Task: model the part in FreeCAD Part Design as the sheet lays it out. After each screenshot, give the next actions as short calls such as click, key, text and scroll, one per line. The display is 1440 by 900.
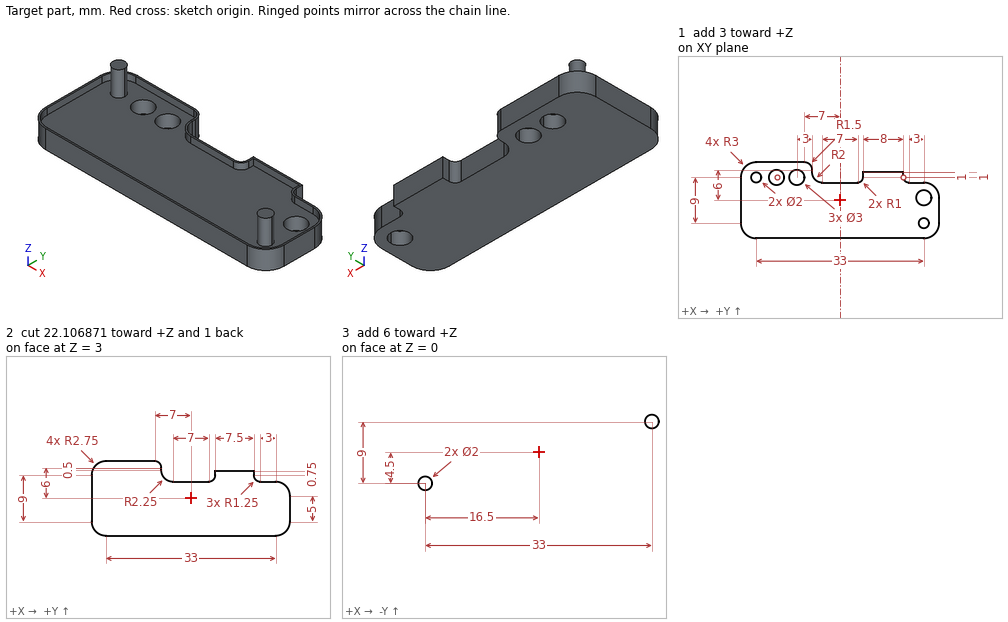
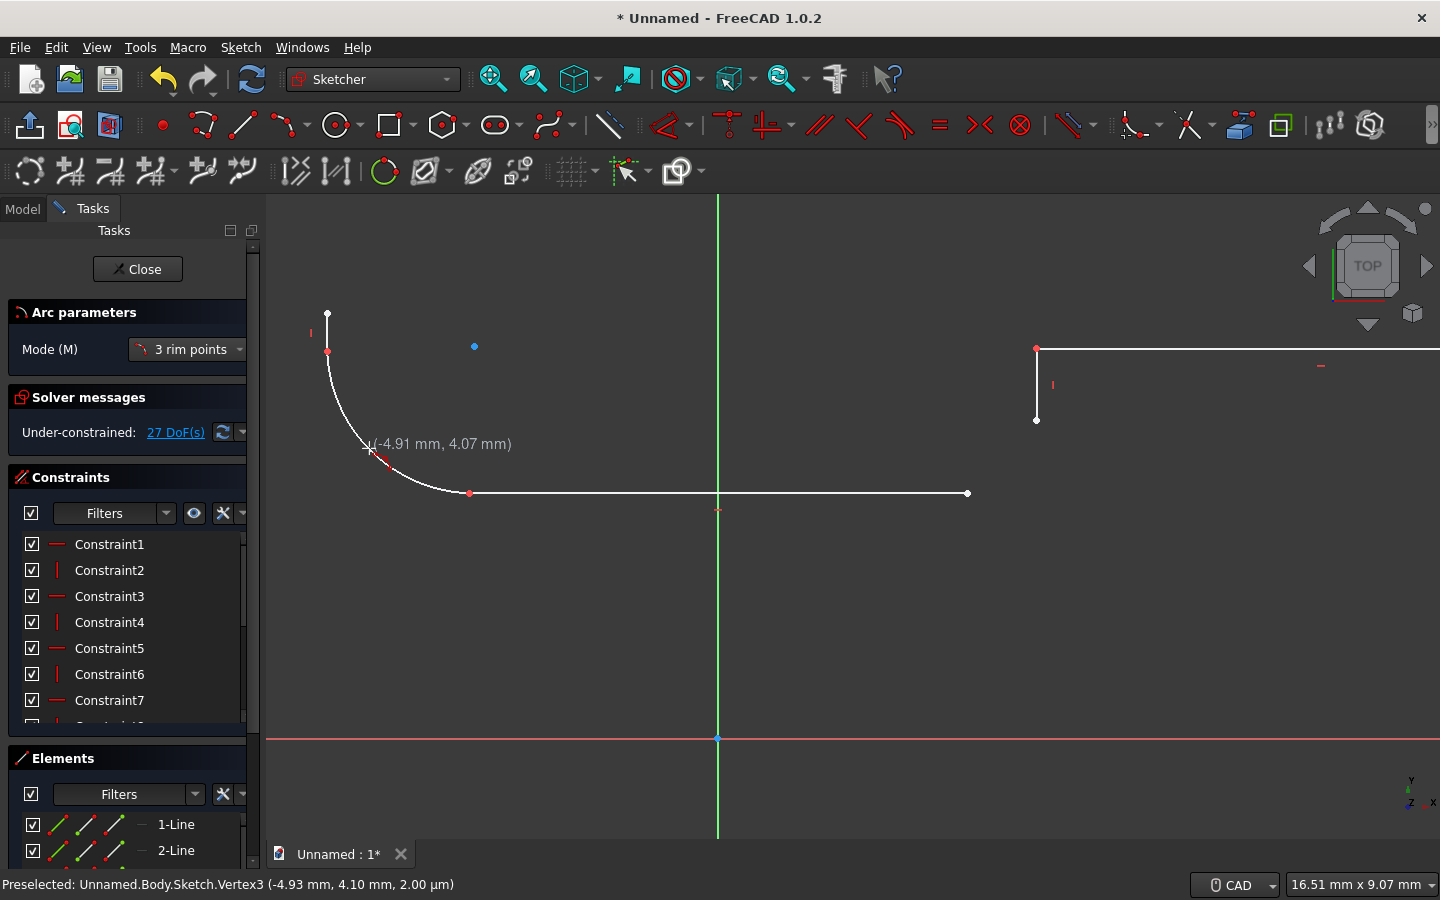
click(327, 314)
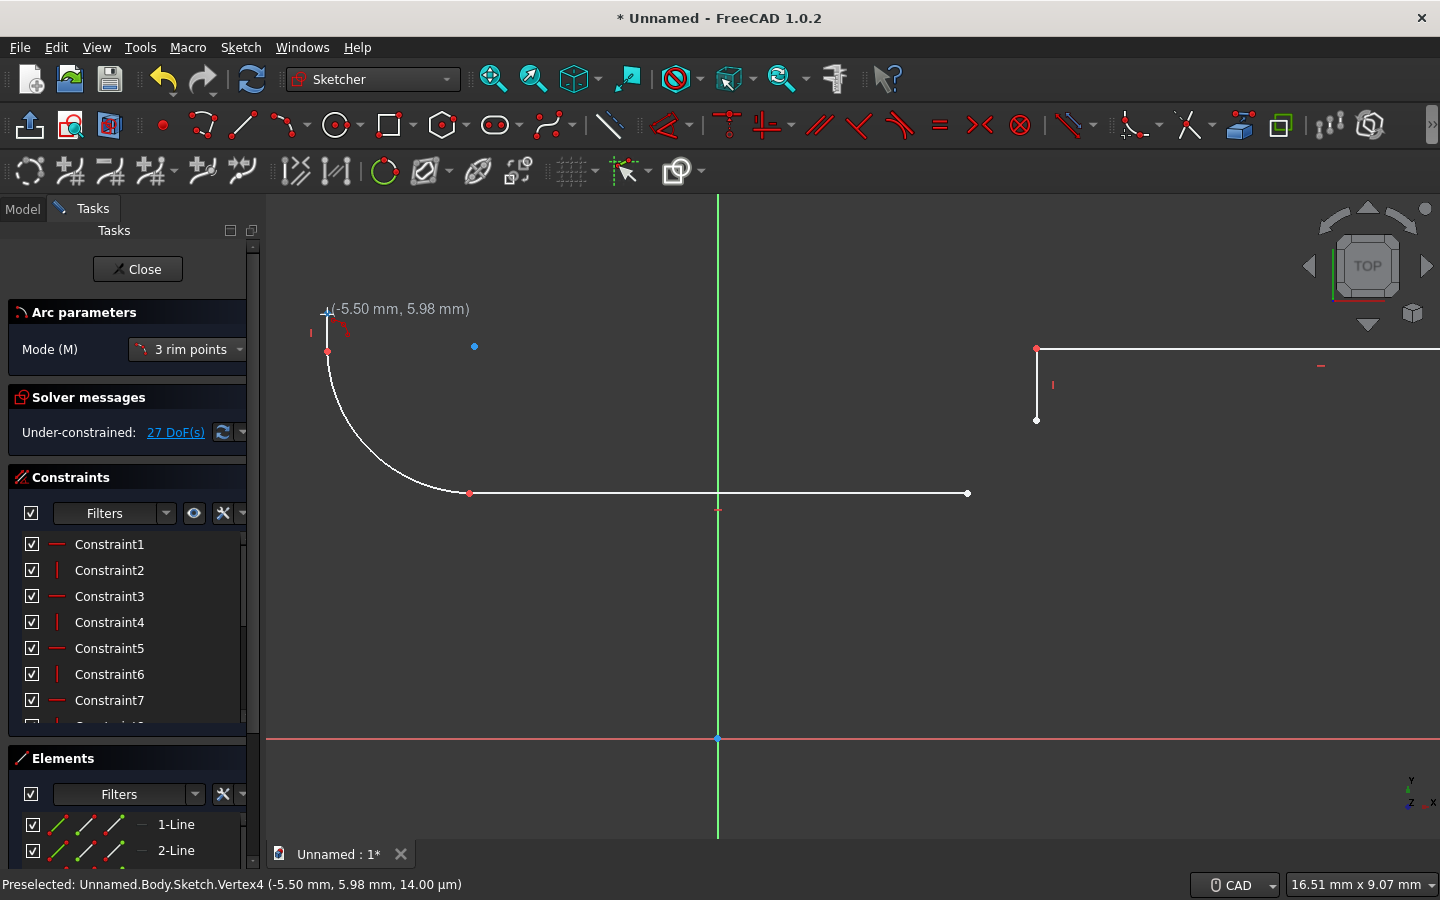
scroll(806, 444, down, 7)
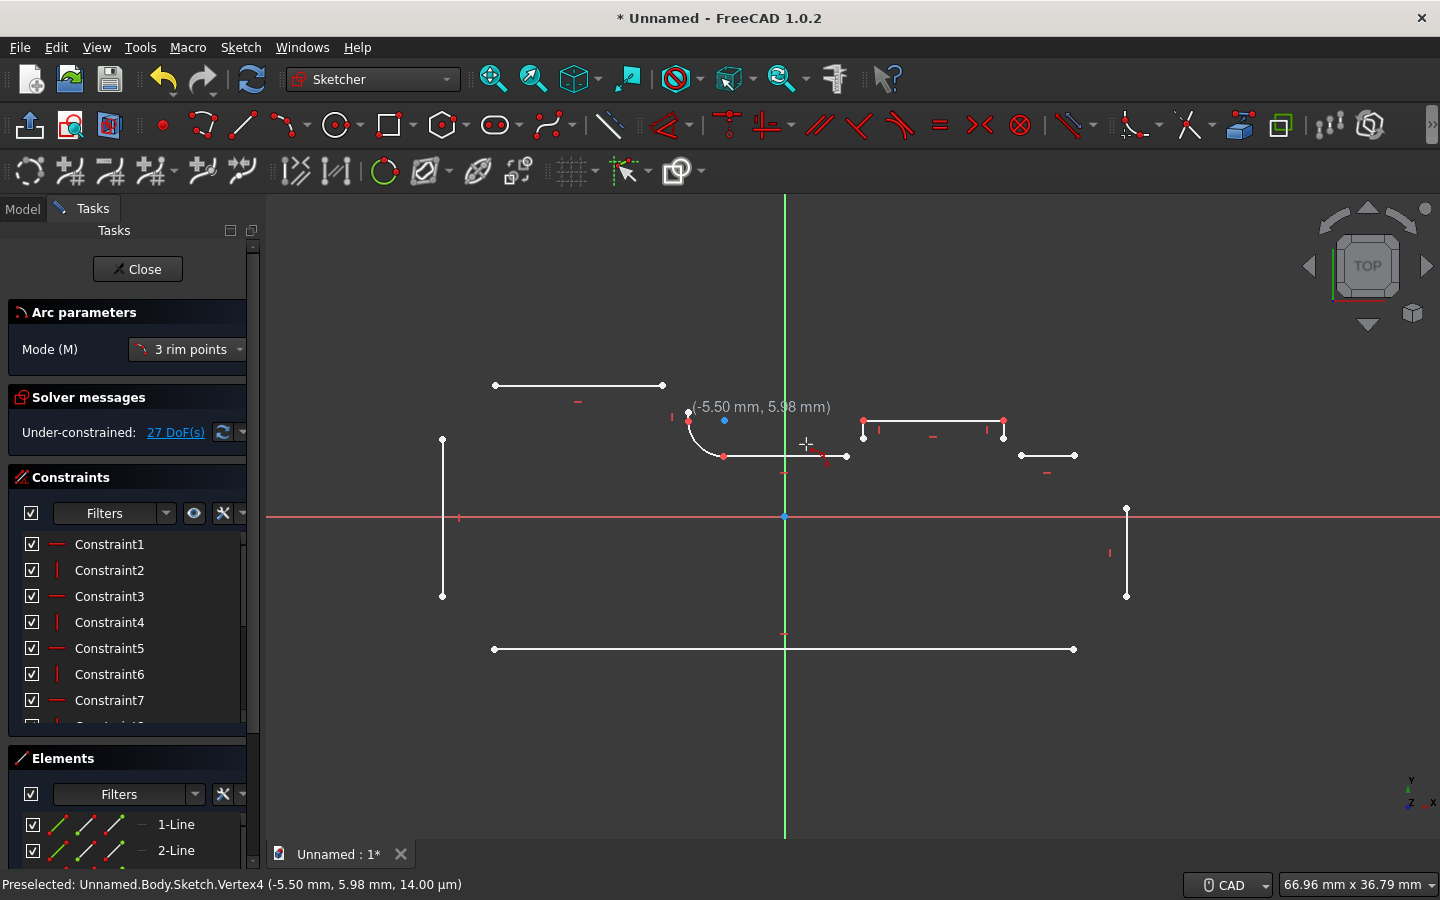
click(662, 386)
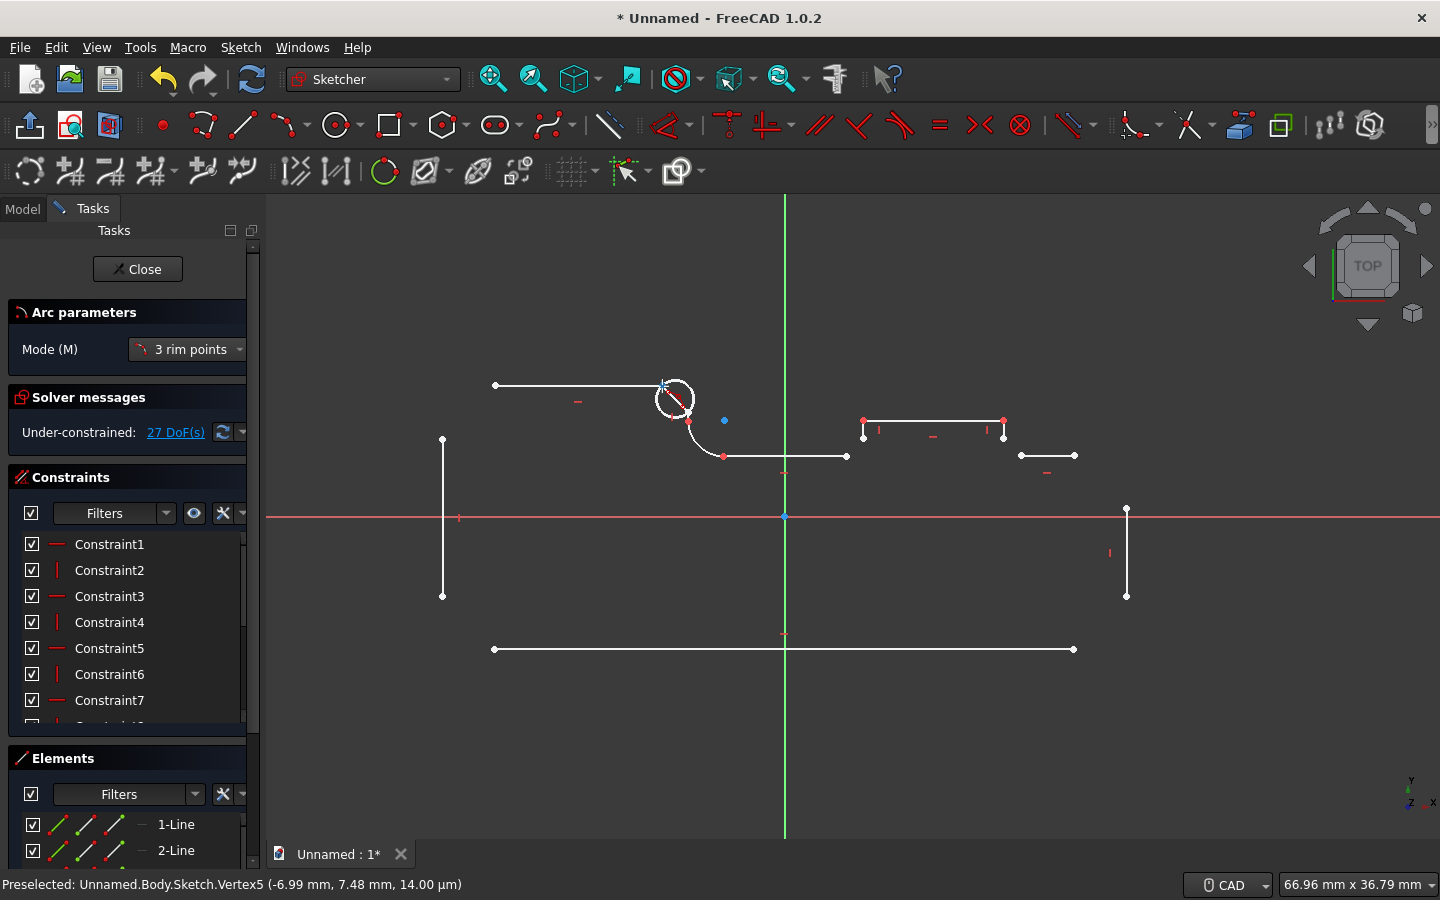
scroll(681, 393, up, 4)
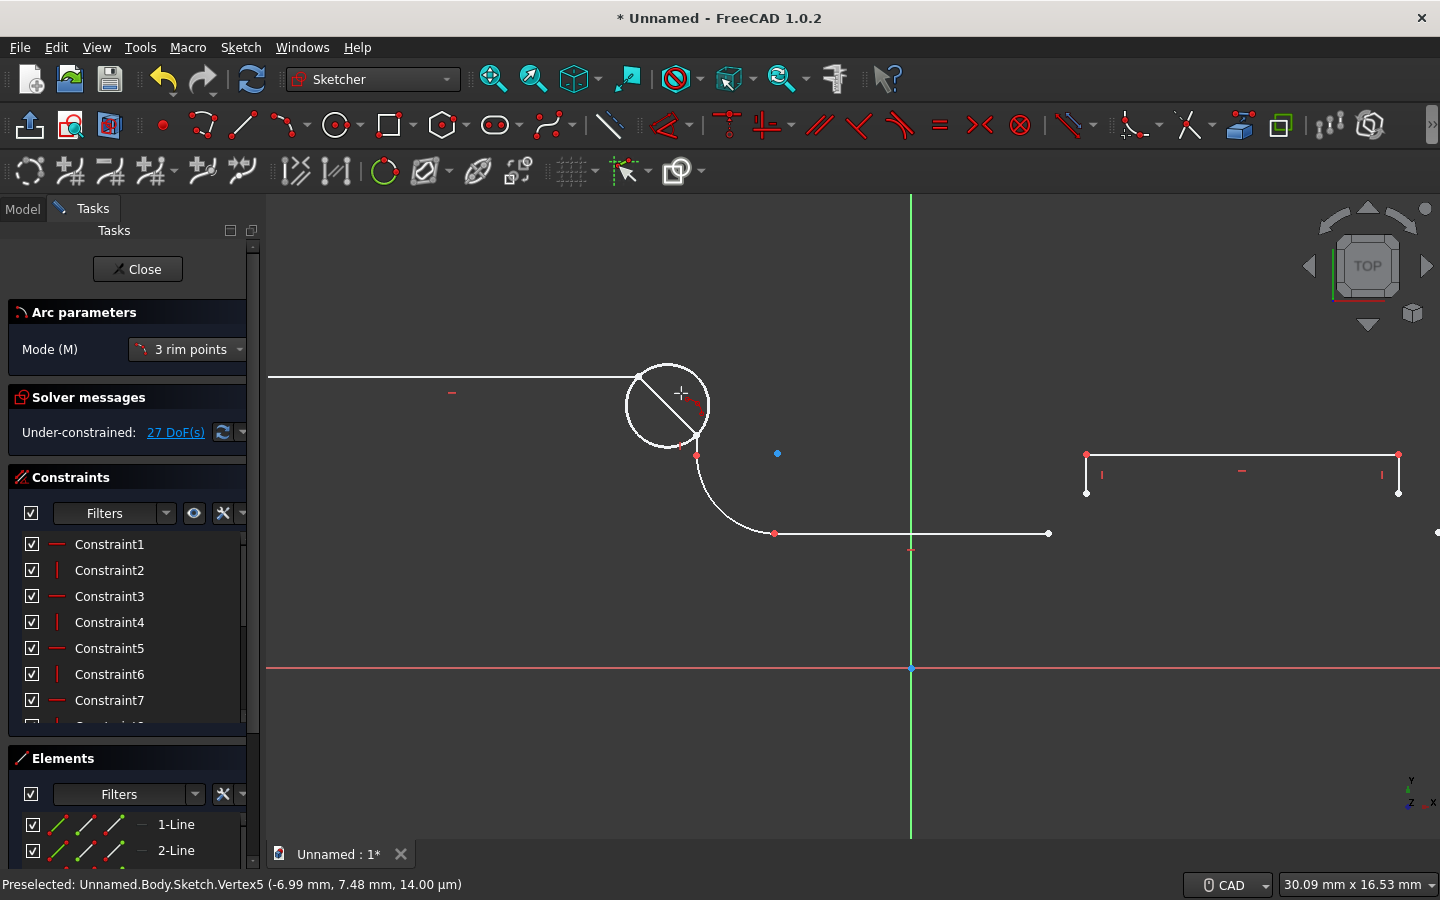
click(679, 393)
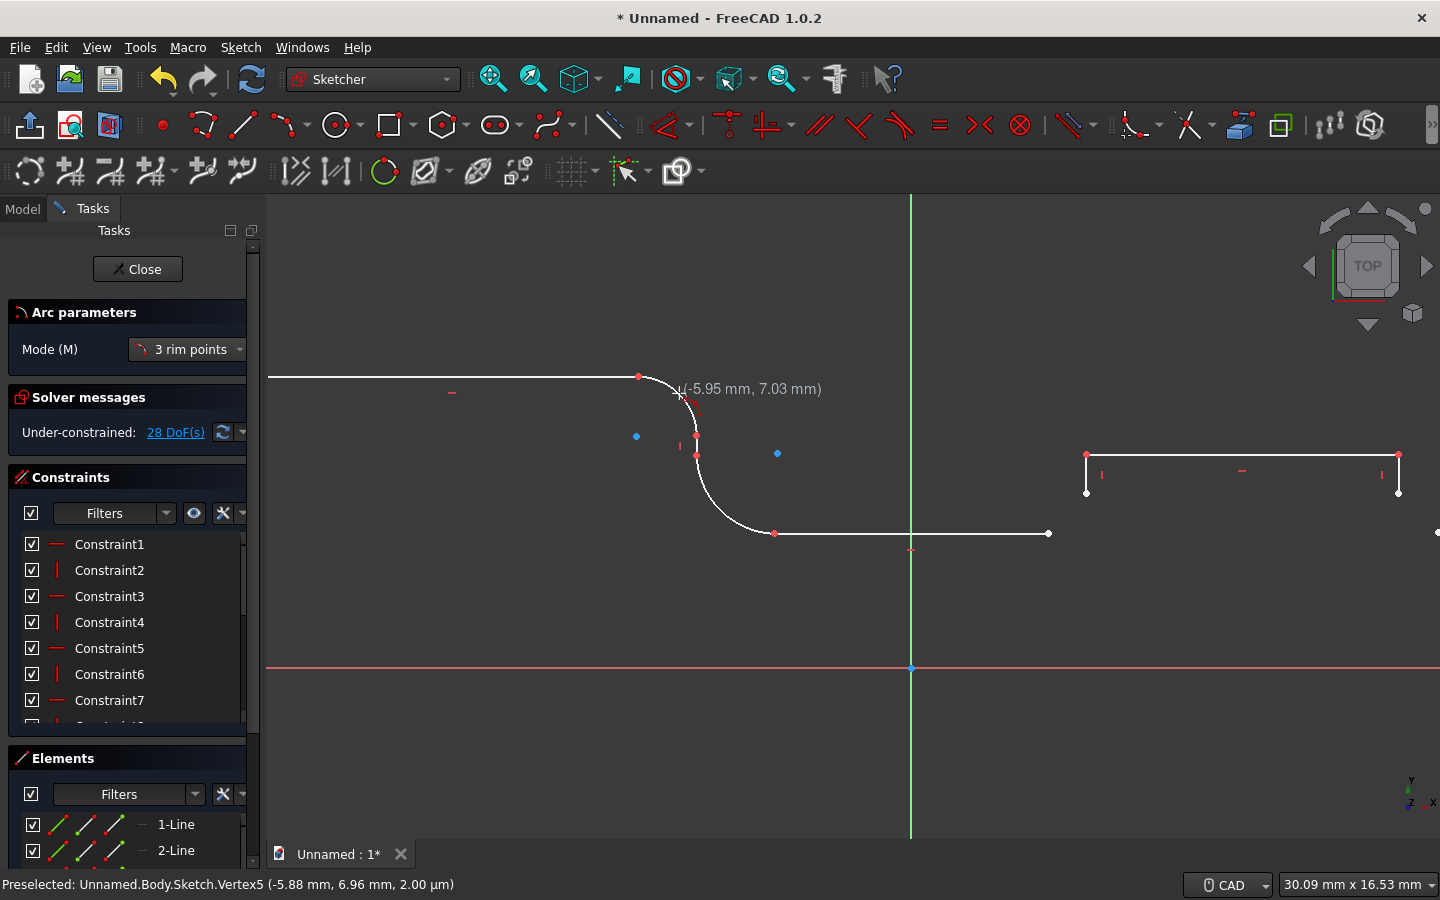
scroll(681, 393, down, 4)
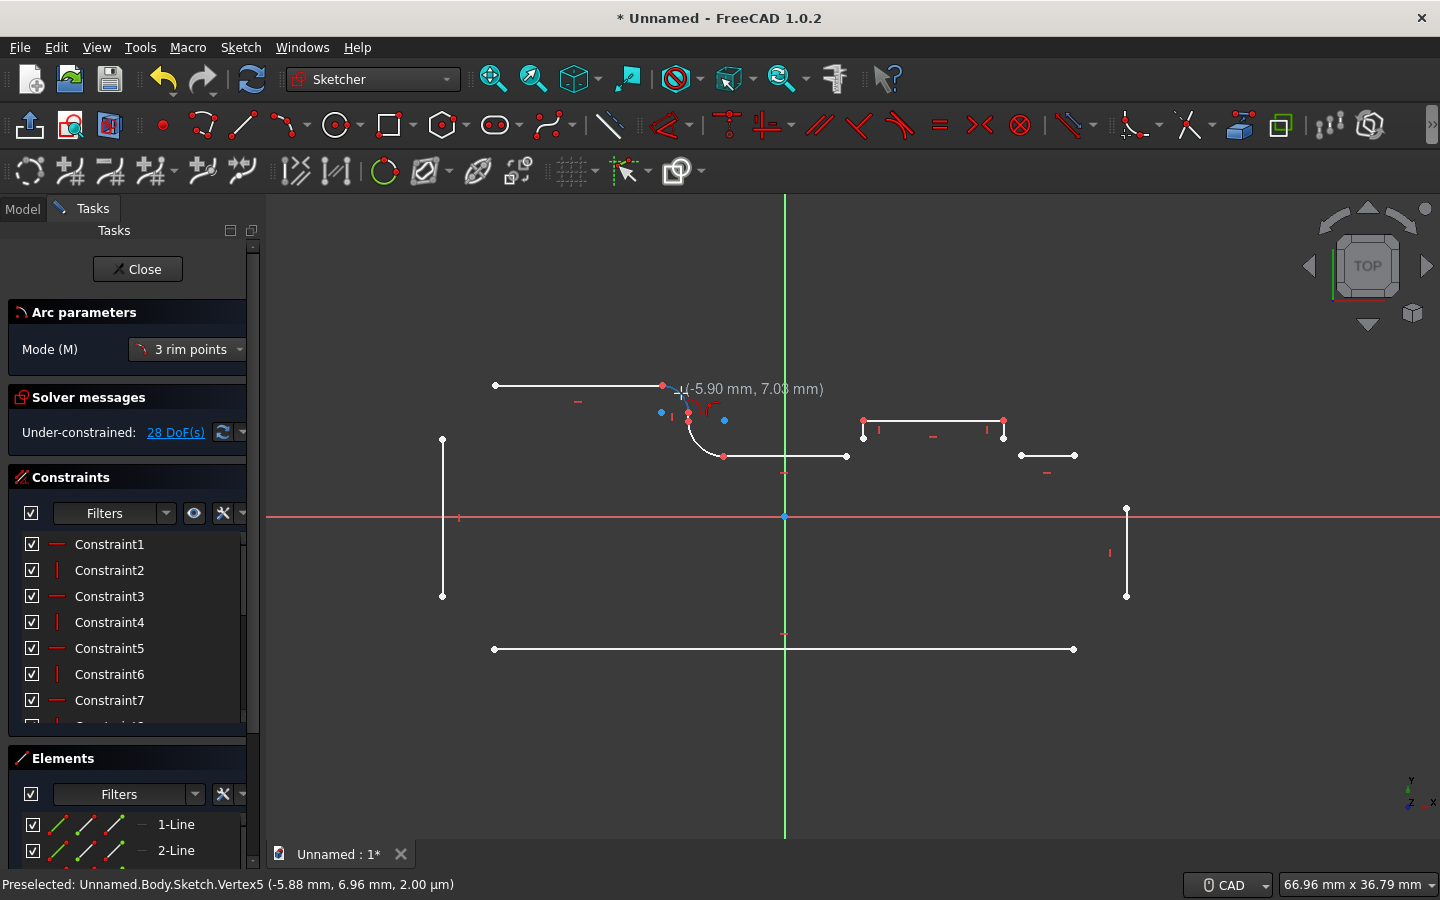
click(495, 386)
click(443, 439)
click(458, 401)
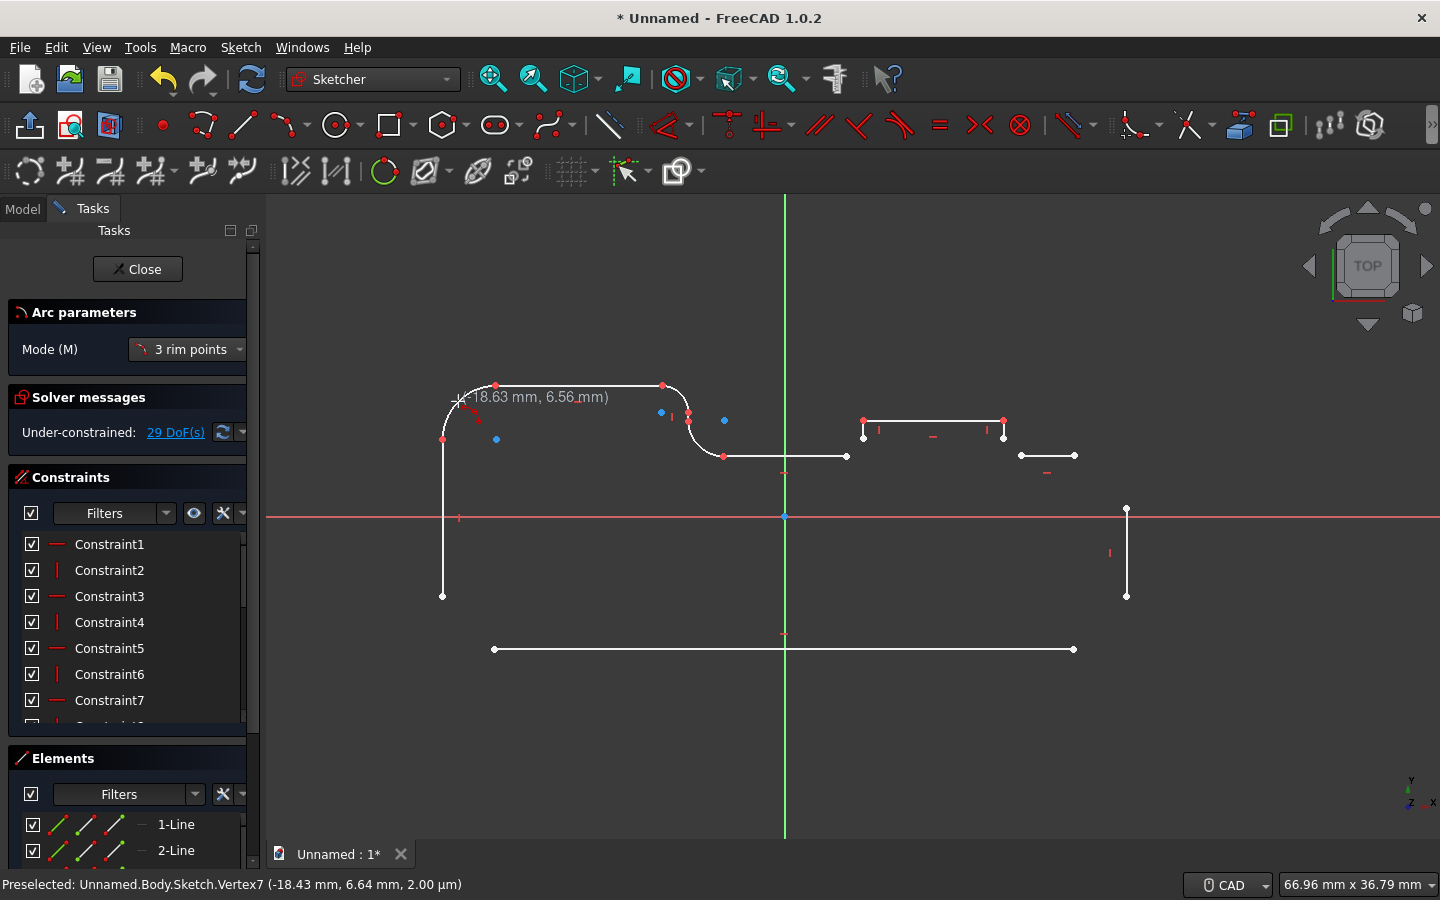
click(443, 596)
click(495, 649)
click(458, 633)